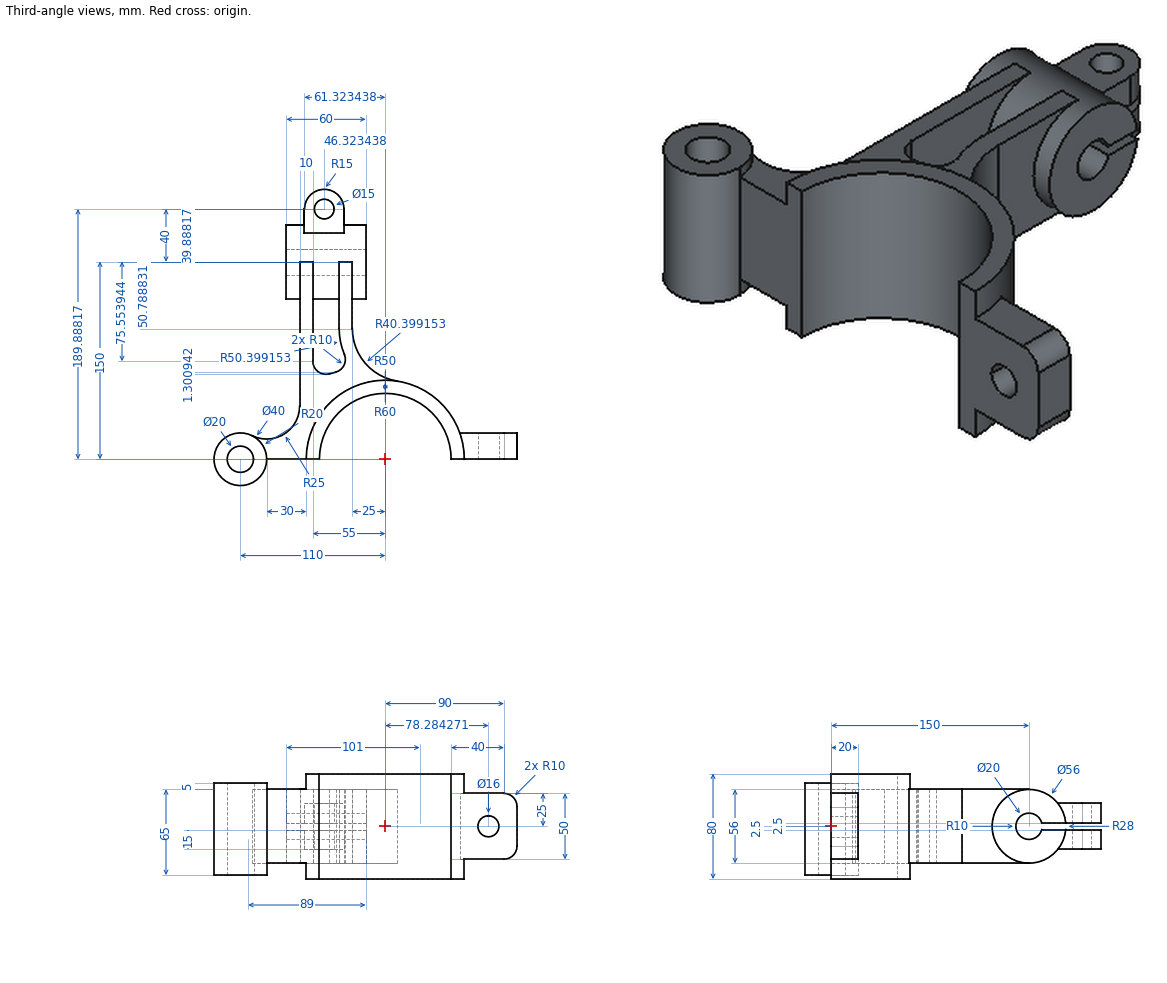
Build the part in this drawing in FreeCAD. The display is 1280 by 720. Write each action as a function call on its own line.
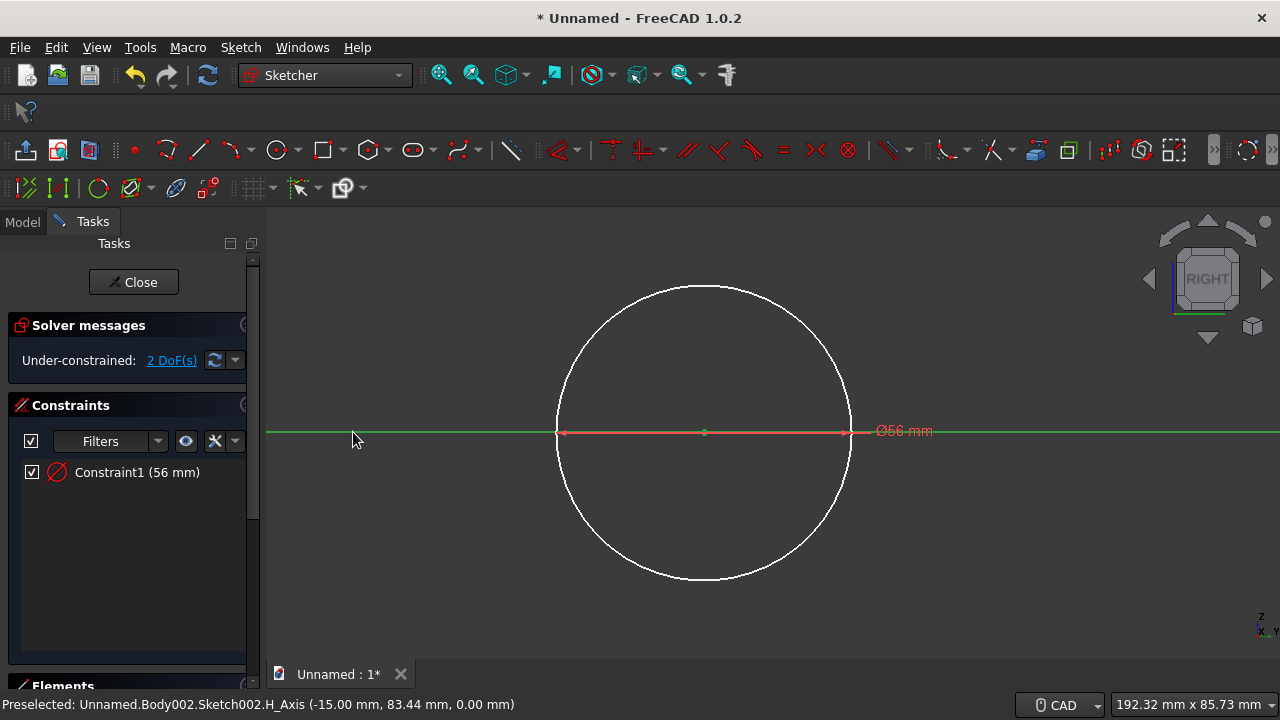
key(c)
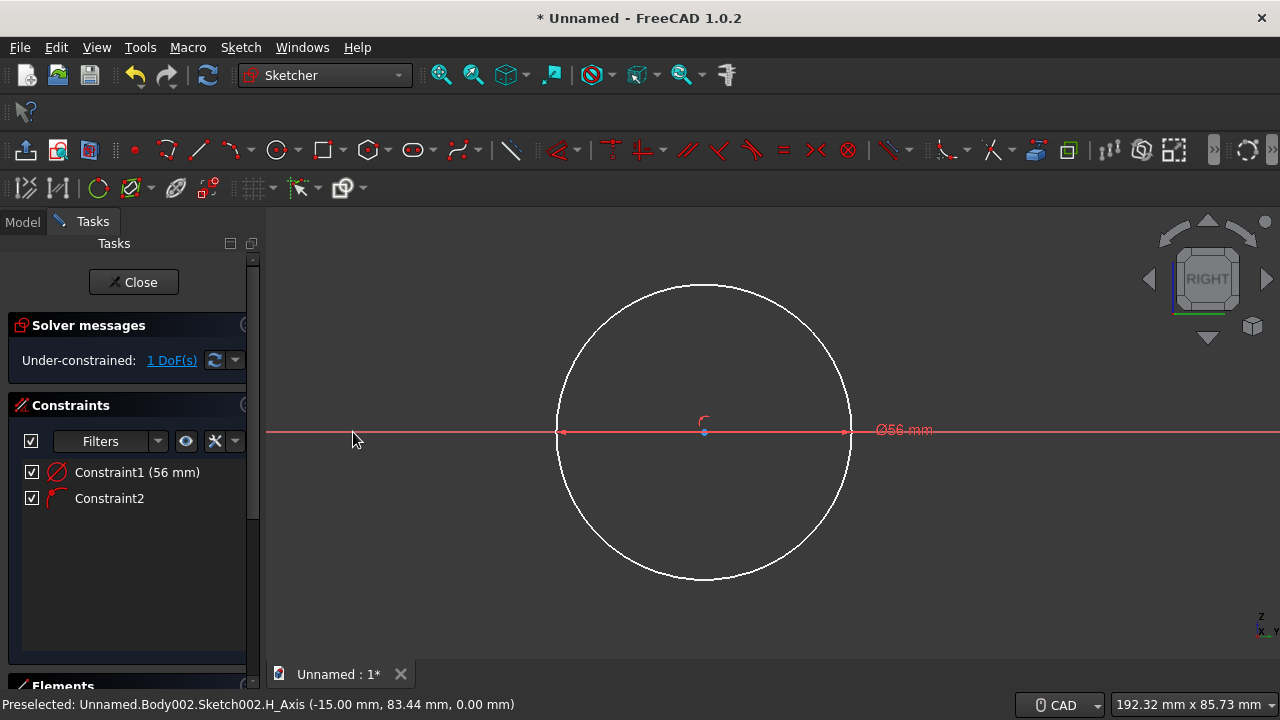
key(d)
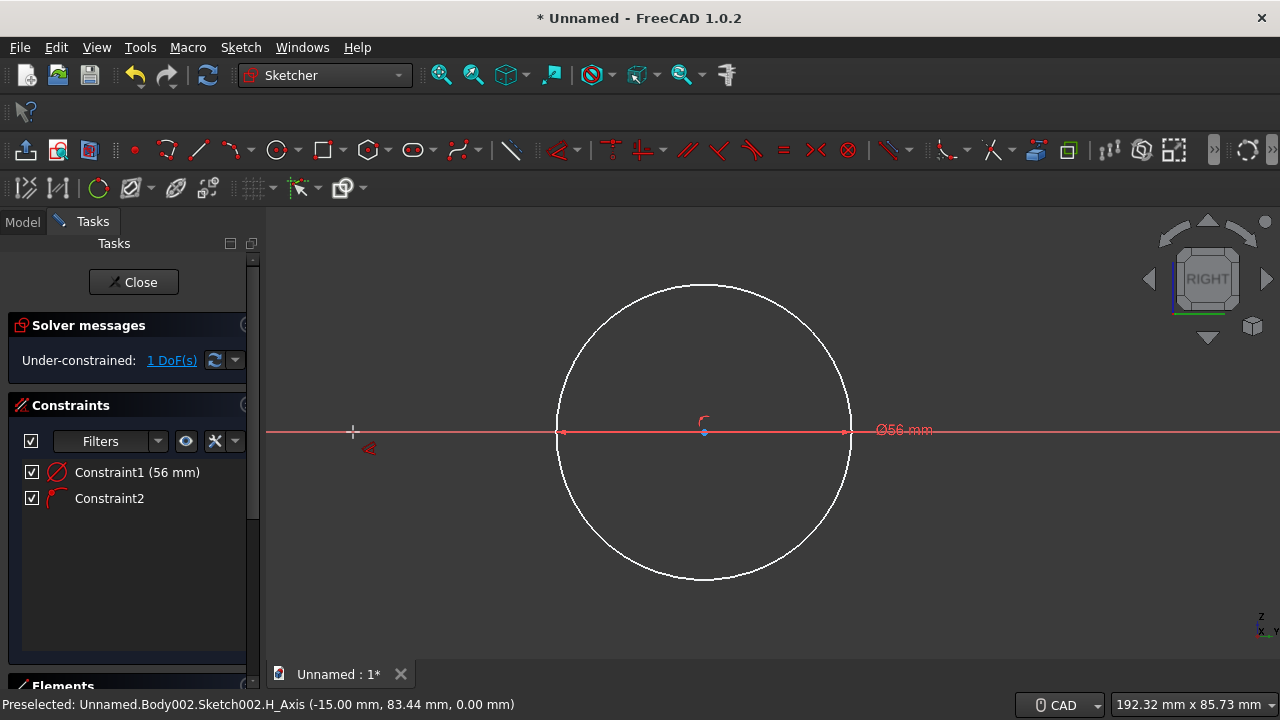
click(704, 432)
click(499, 466)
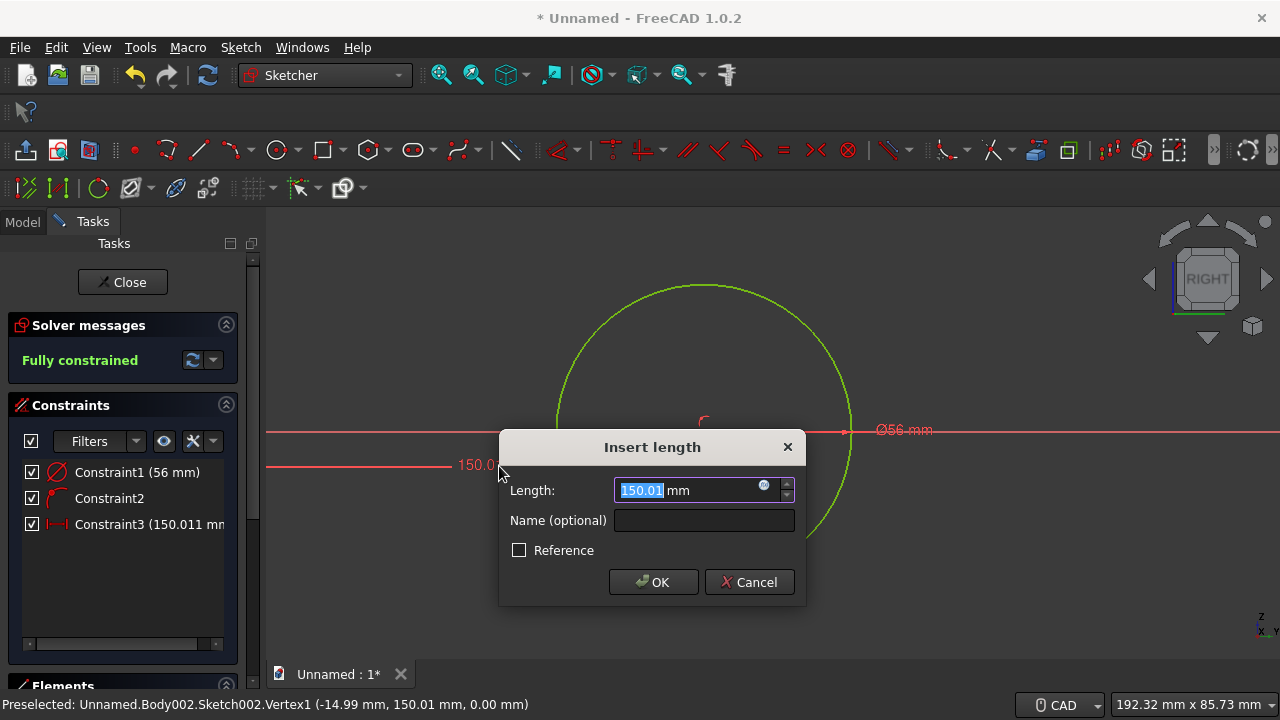
text(150)
key(Return)
key(Escape)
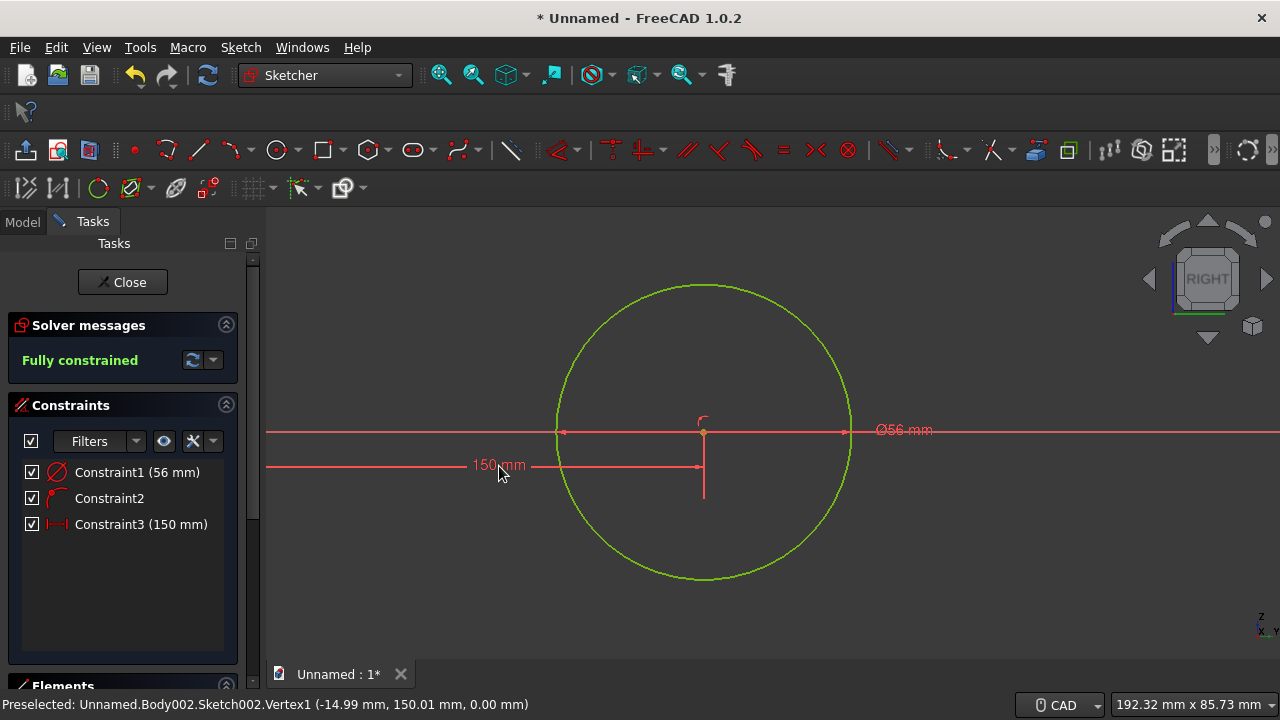
click(123, 282)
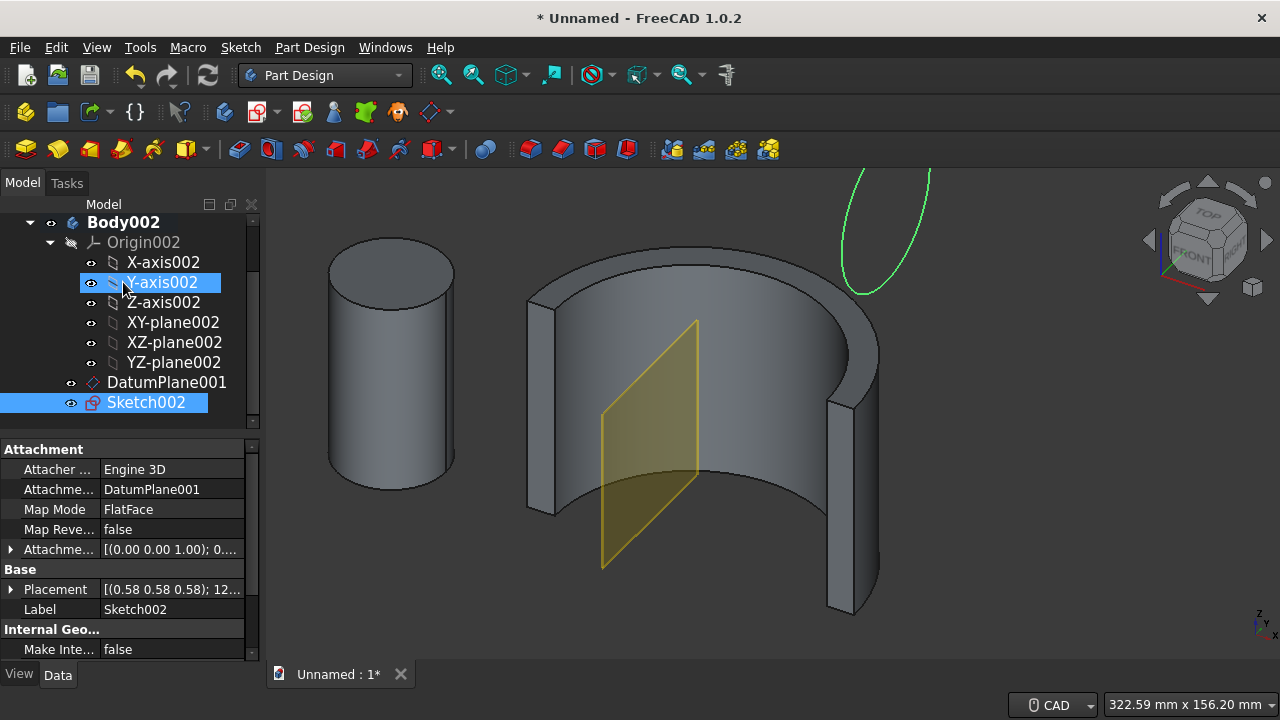
click(26, 150)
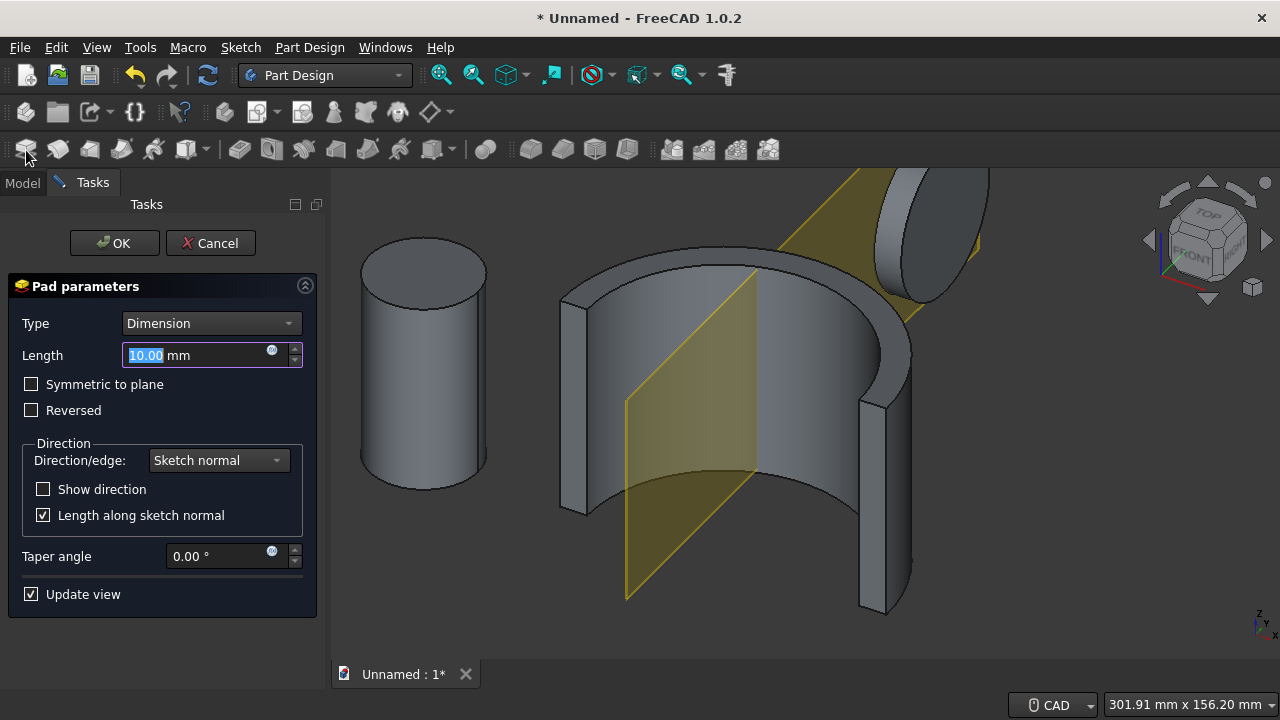
text(60)
key(Tab)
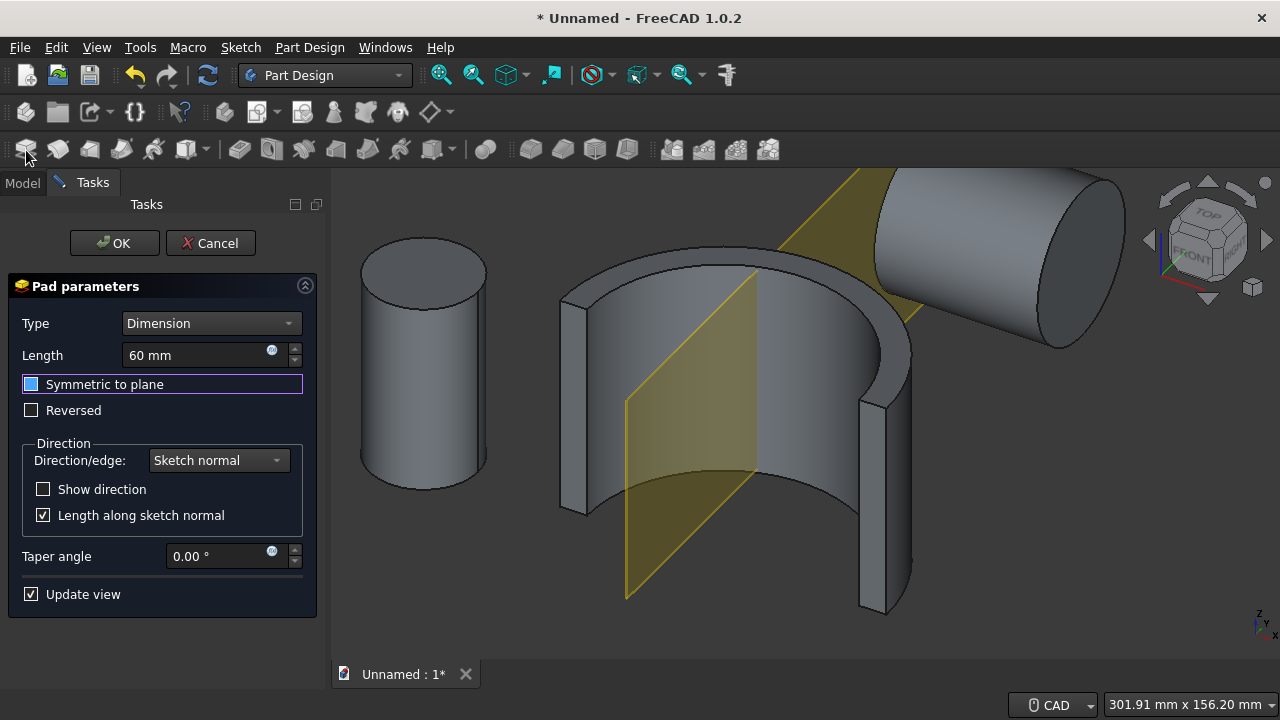
click(30, 410)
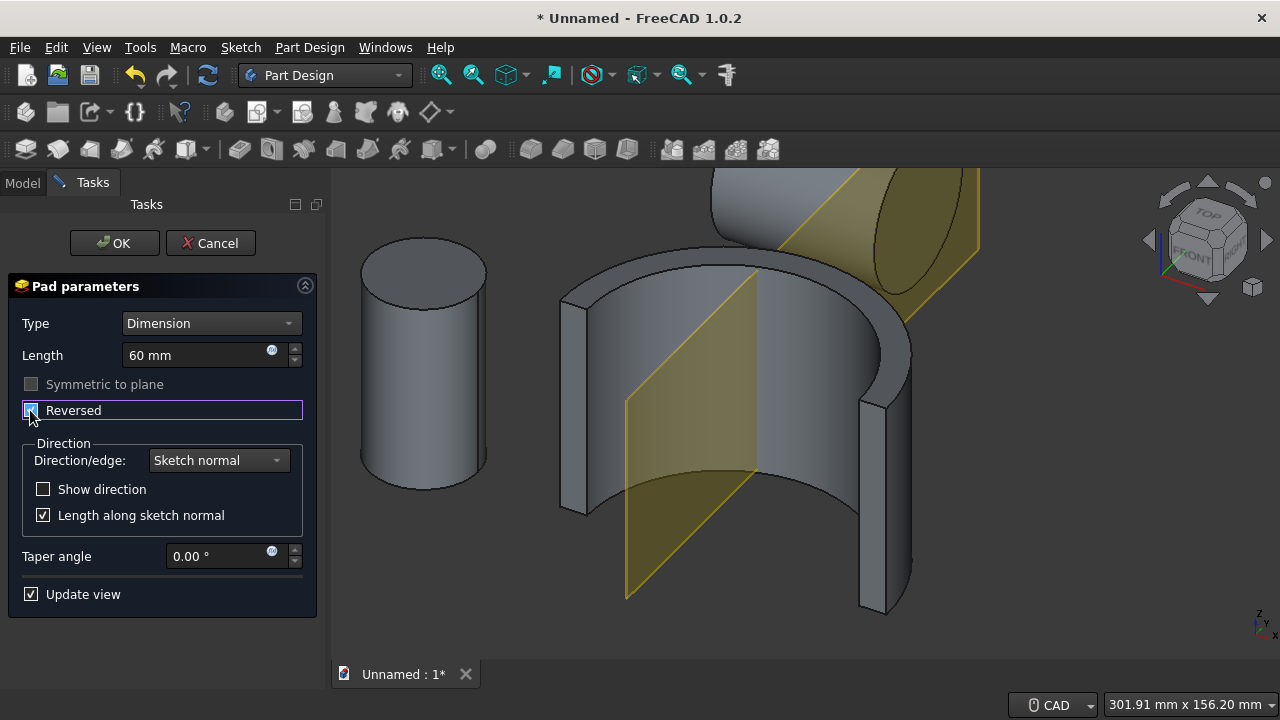
click(115, 243)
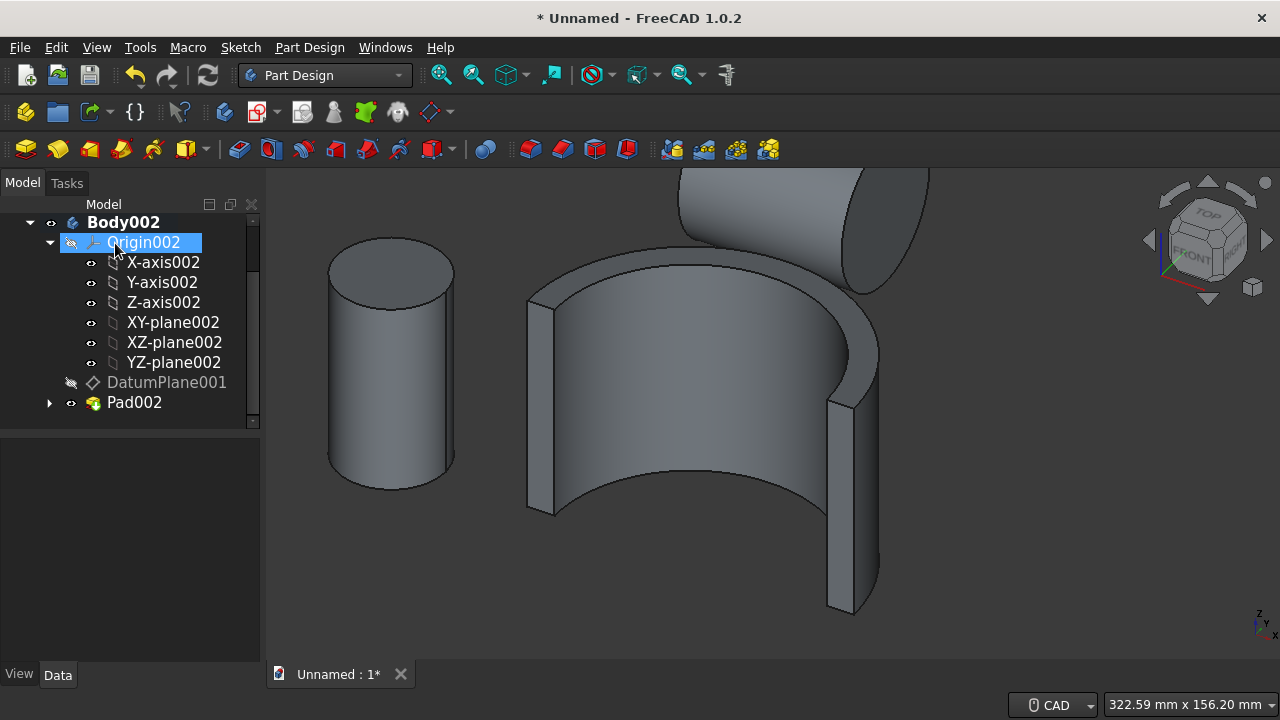
key(v)
key(f)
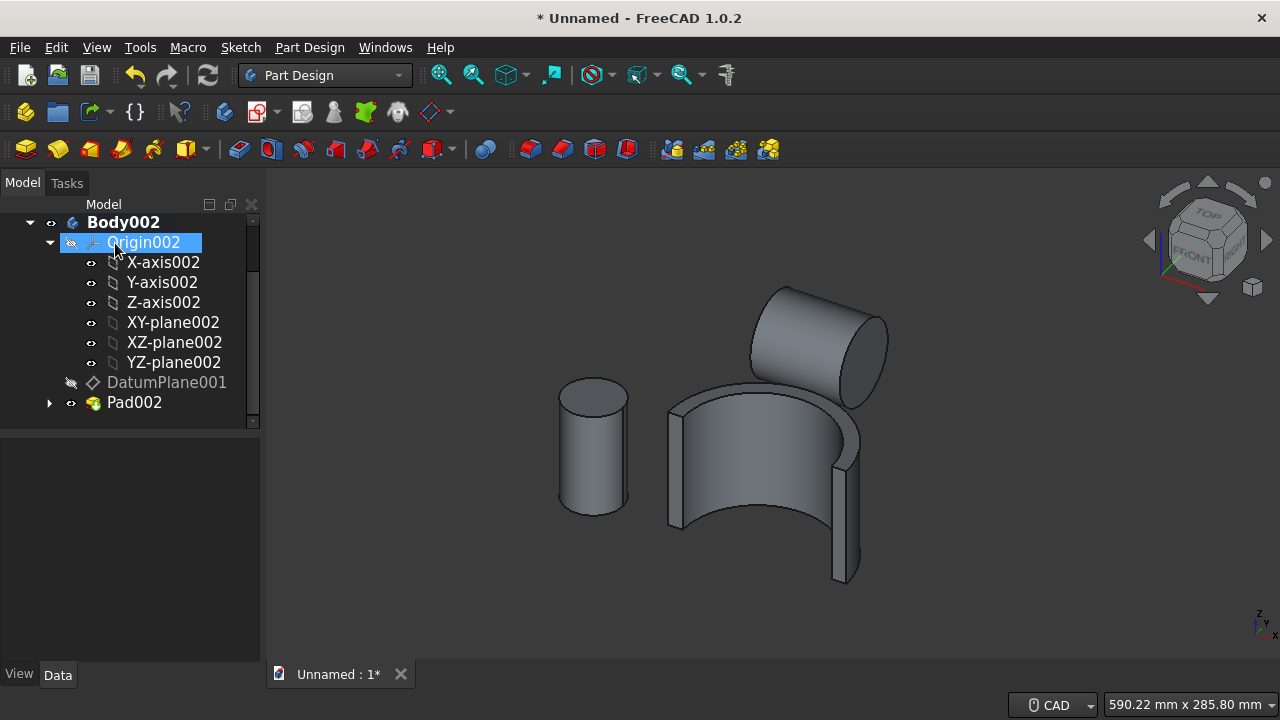
scroll(120, 318, down, 3)